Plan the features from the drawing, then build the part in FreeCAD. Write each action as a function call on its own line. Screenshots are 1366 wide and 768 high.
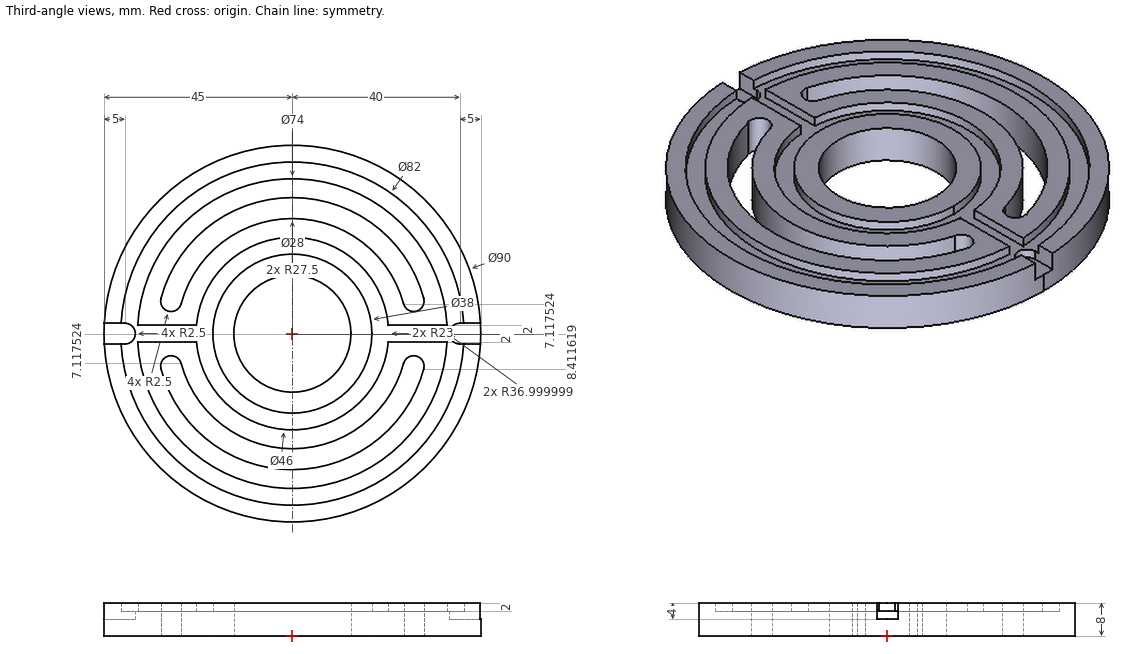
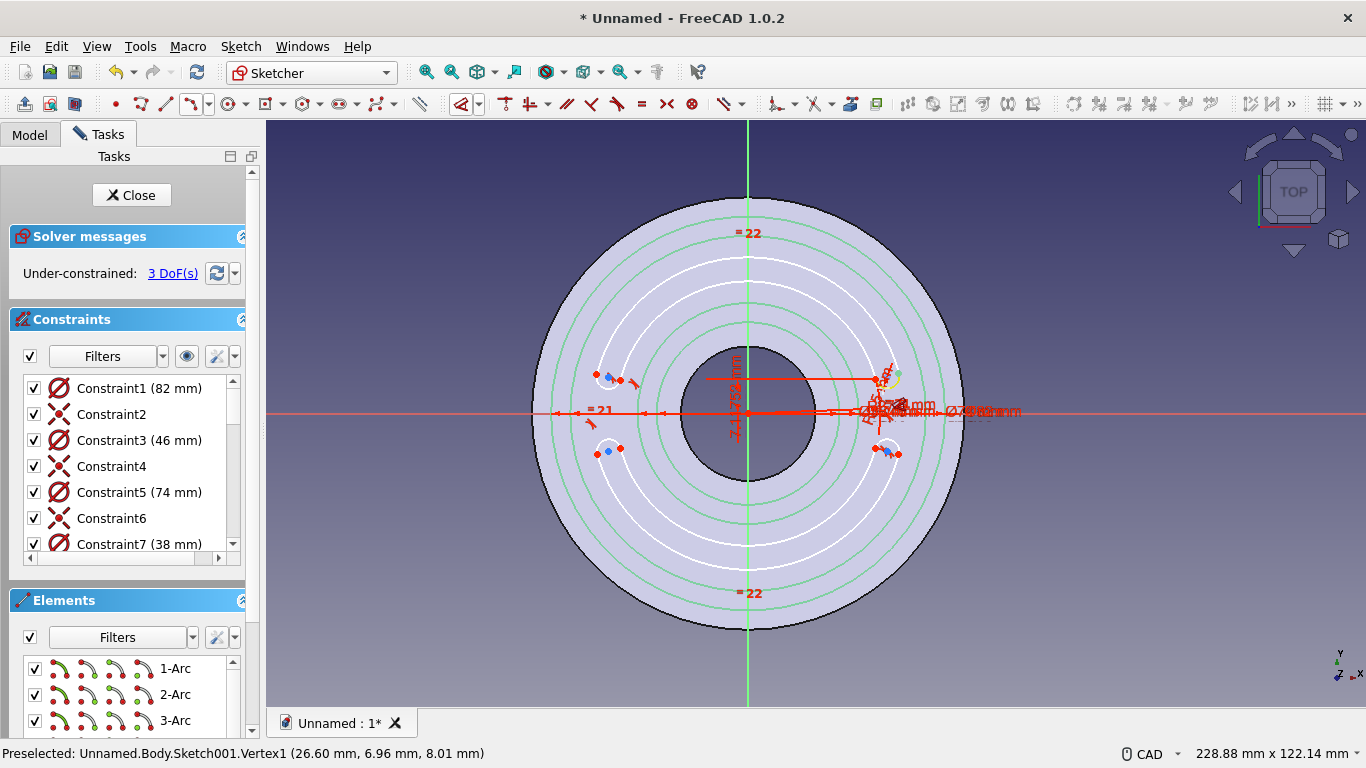
click(620, 380)
click(586, 397)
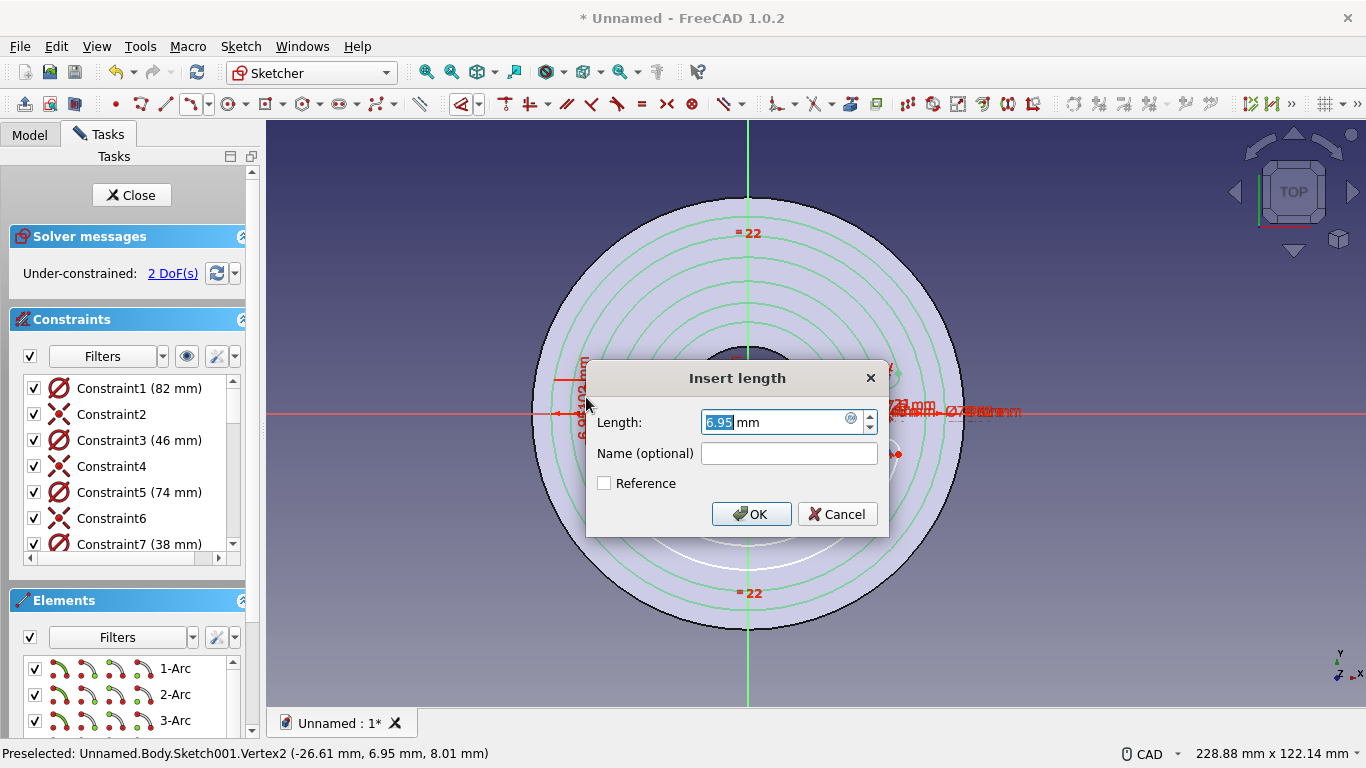
text(7.117524)
key(Return)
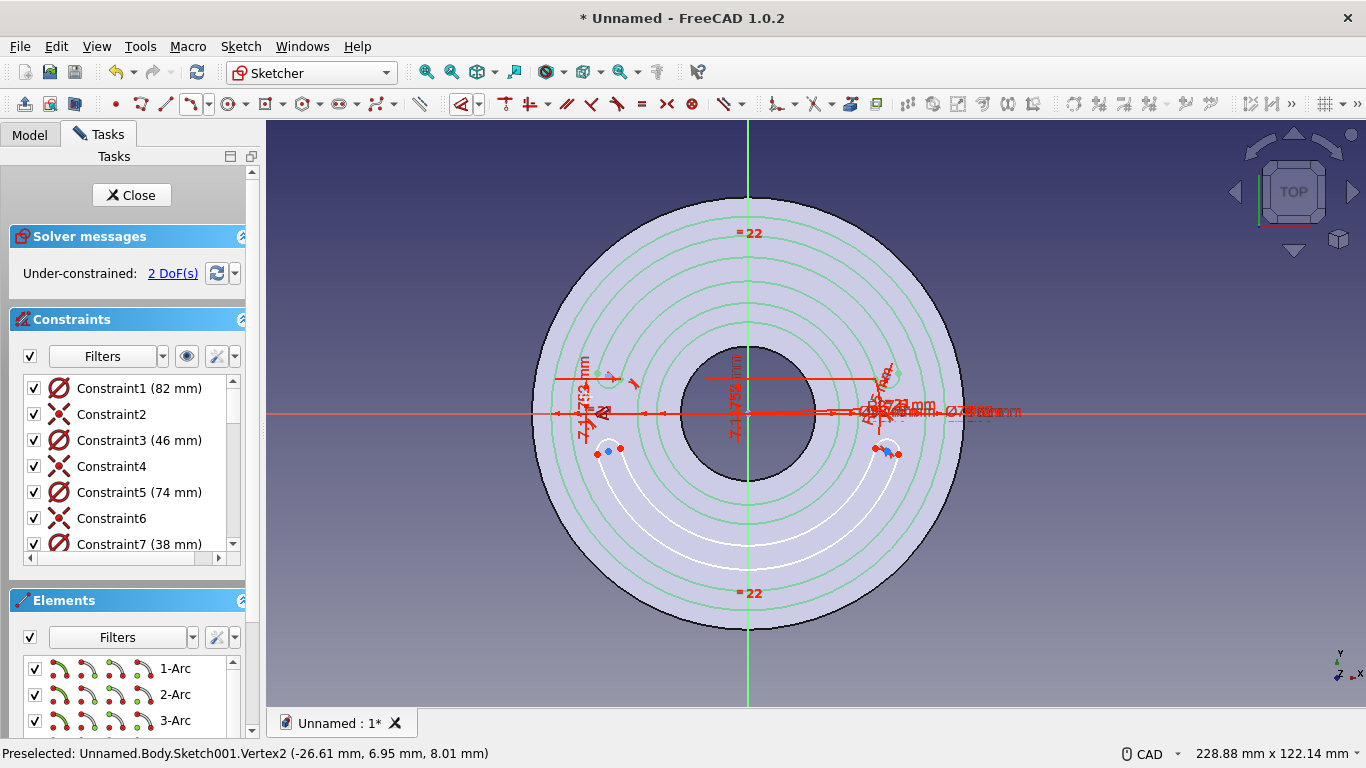
click(621, 448)
click(587, 431)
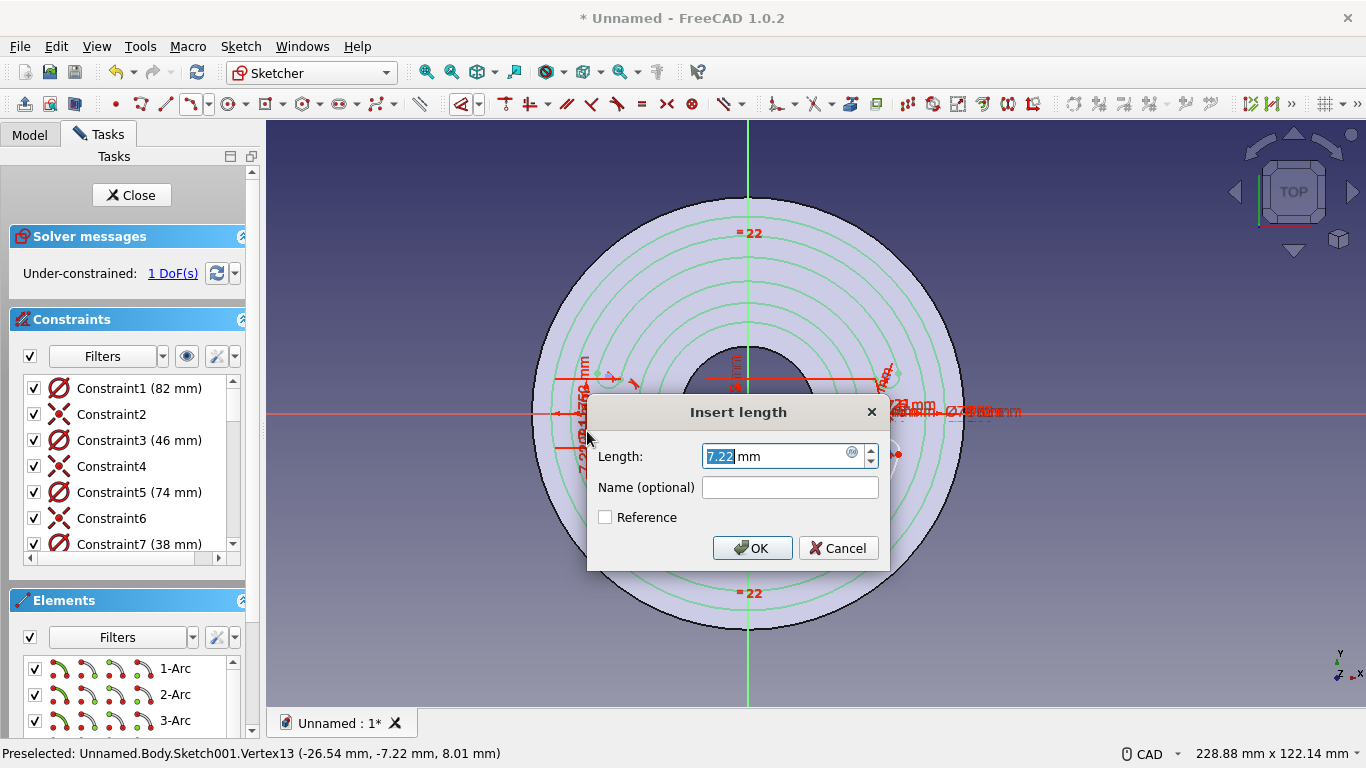
text(7.117524)
key(Return)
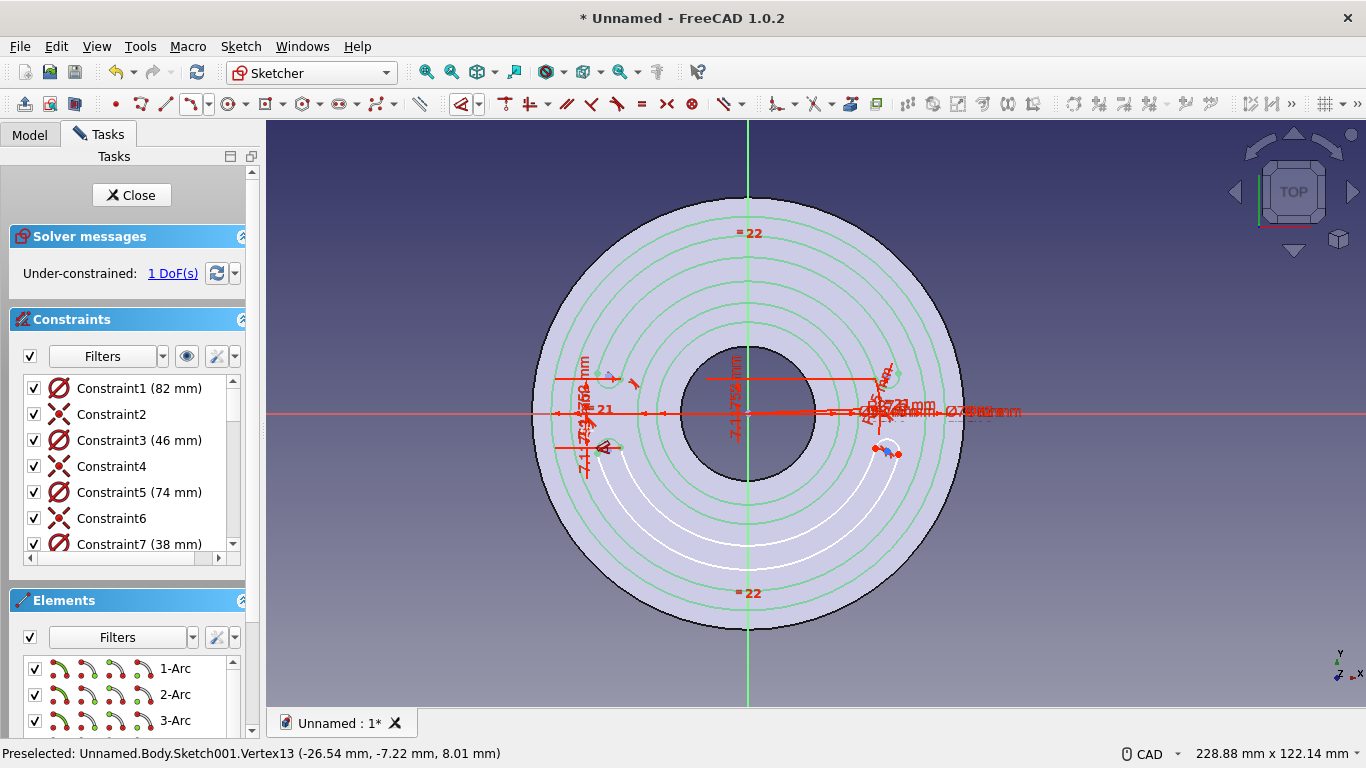
click(899, 455)
click(714, 434)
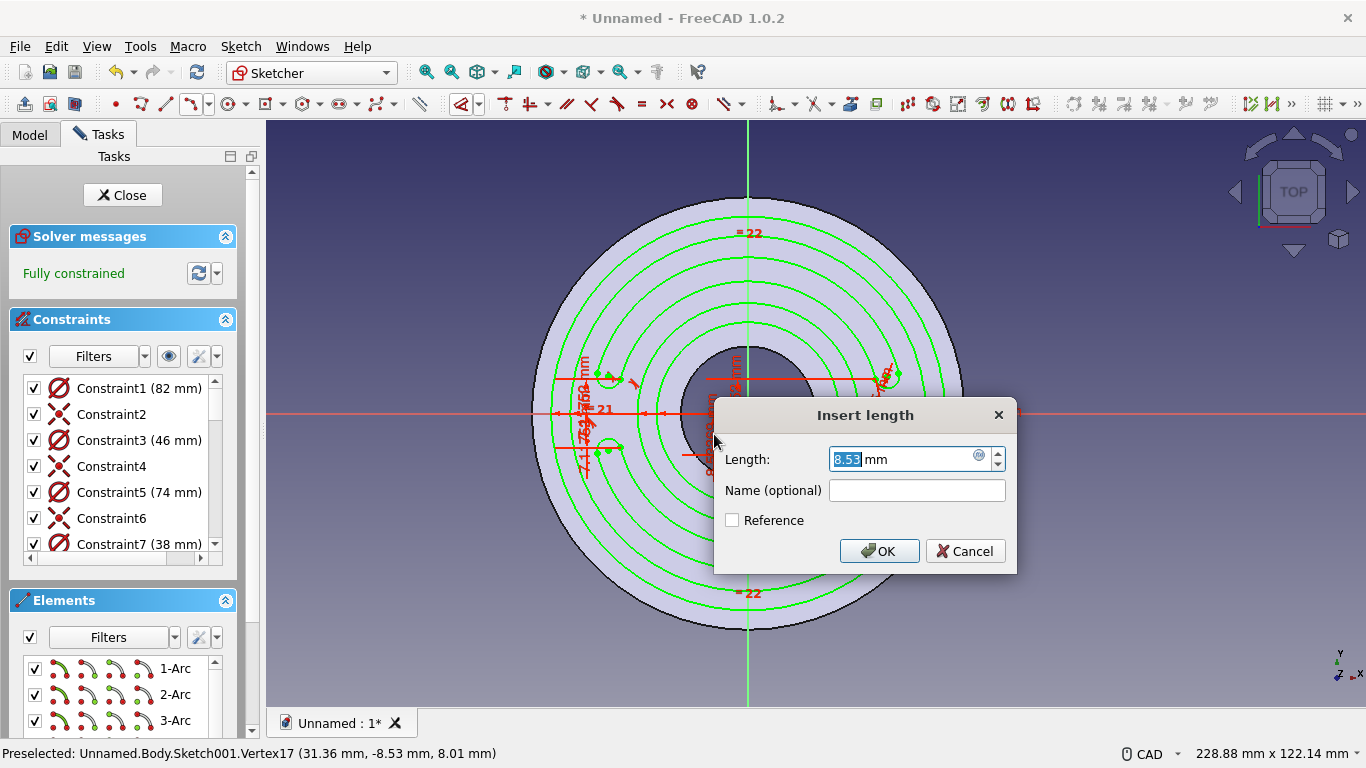
text(8.411619)
key(Return)
key(Escape)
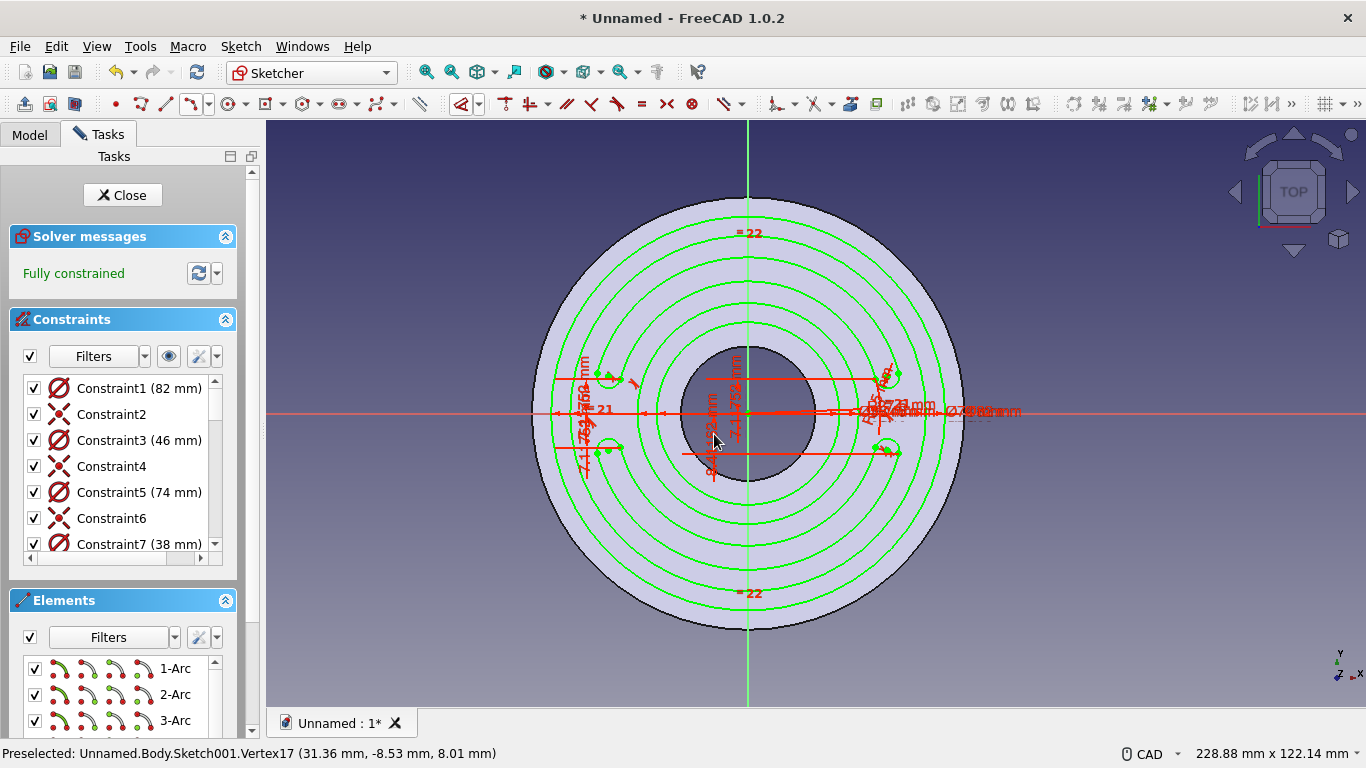
click(123, 195)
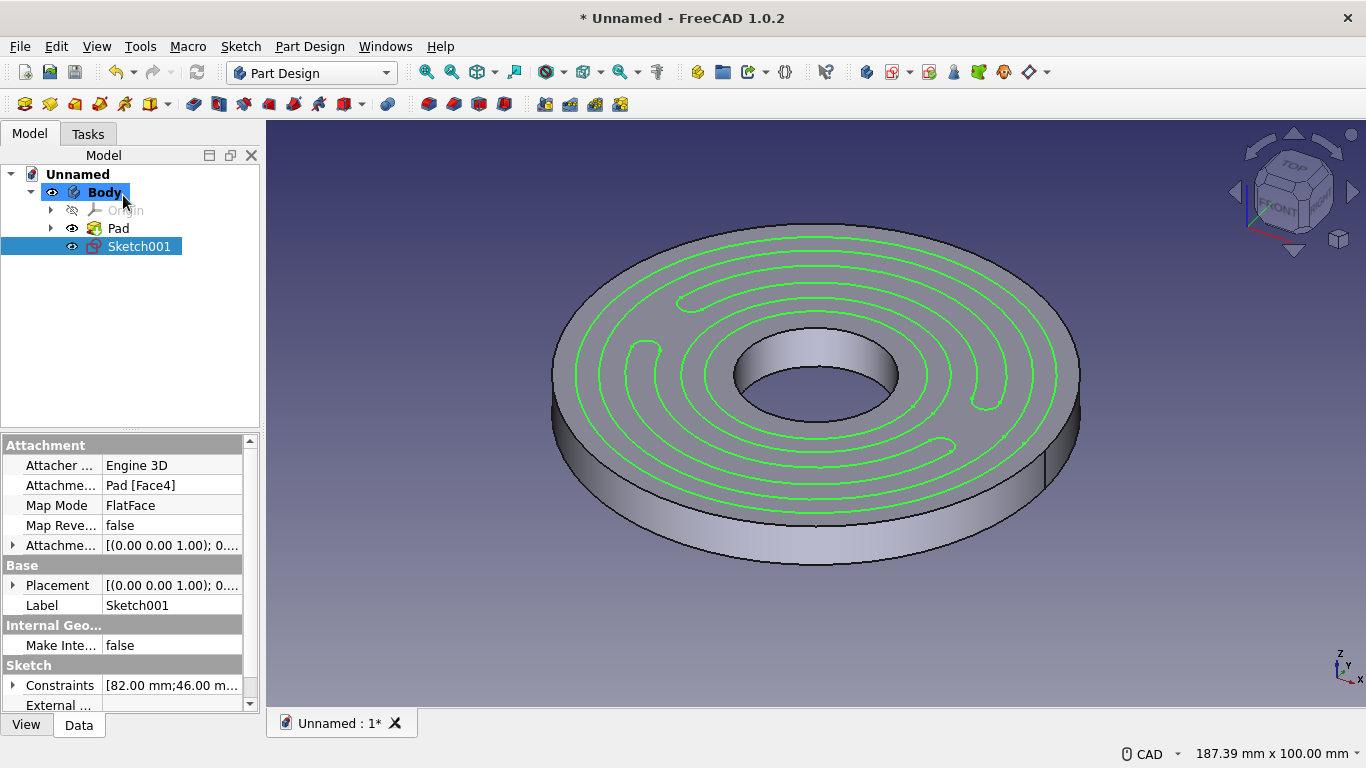
click(194, 104)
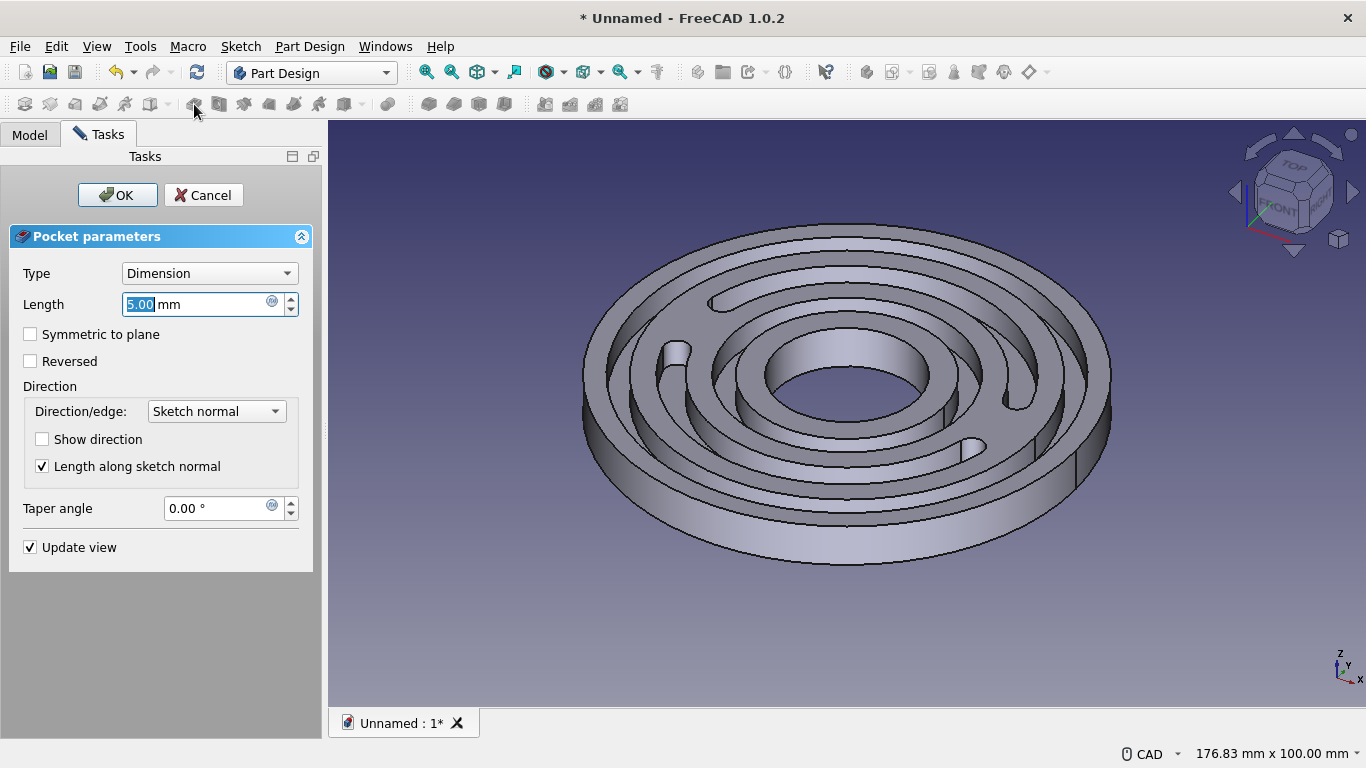
text(2)
key(Tab)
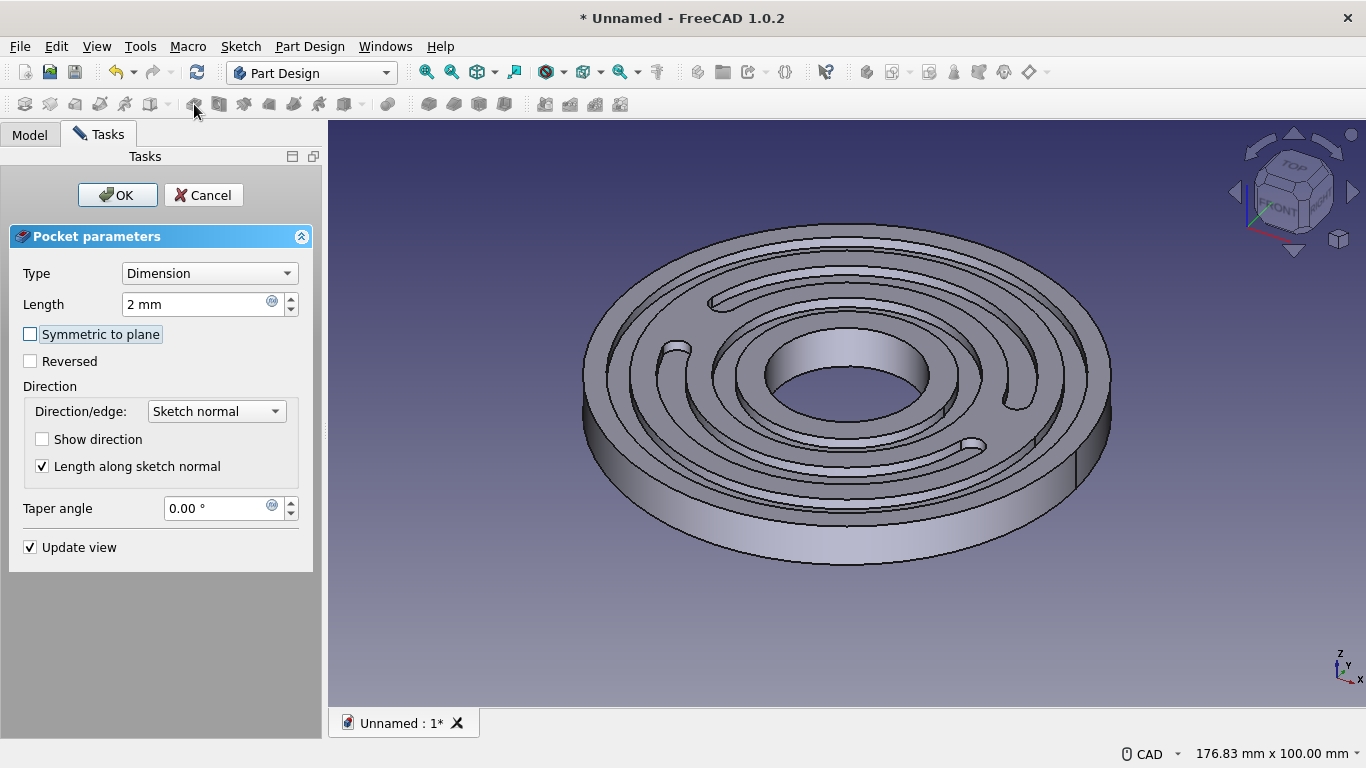
click(118, 195)